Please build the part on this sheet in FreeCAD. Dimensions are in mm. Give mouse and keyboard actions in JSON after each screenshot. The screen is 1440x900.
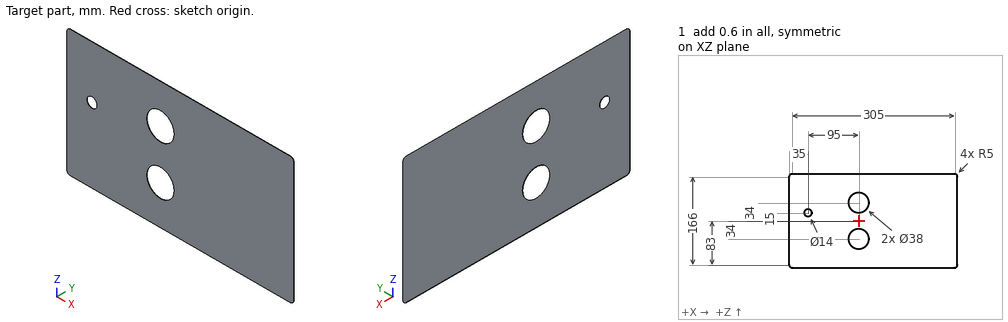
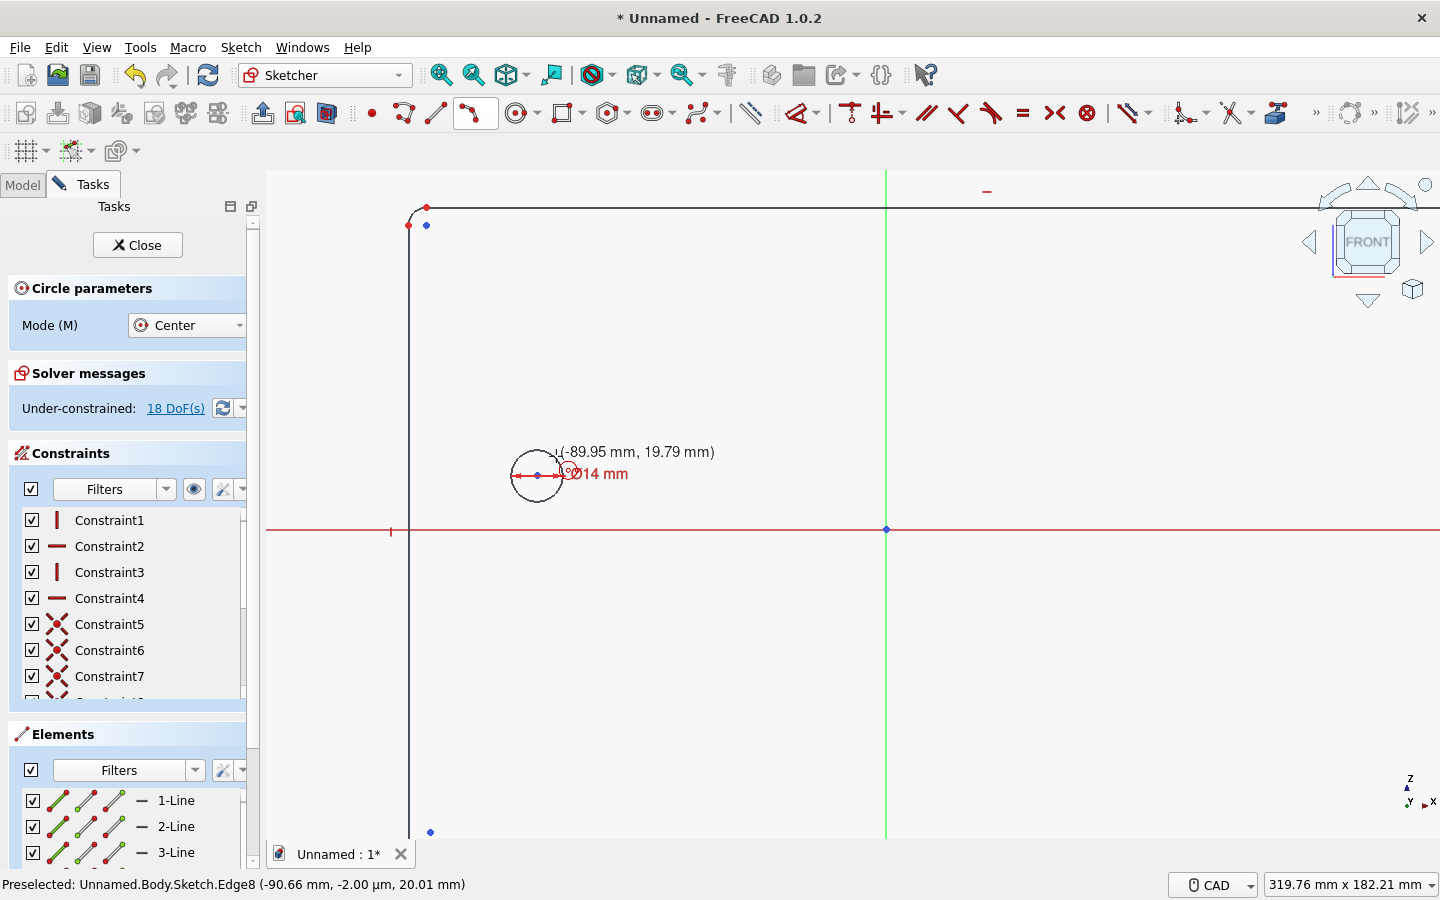
{"action": "left_click", "coordinate": [886, 405]}
{"action": "mouse_move", "coordinate": [936, 355]}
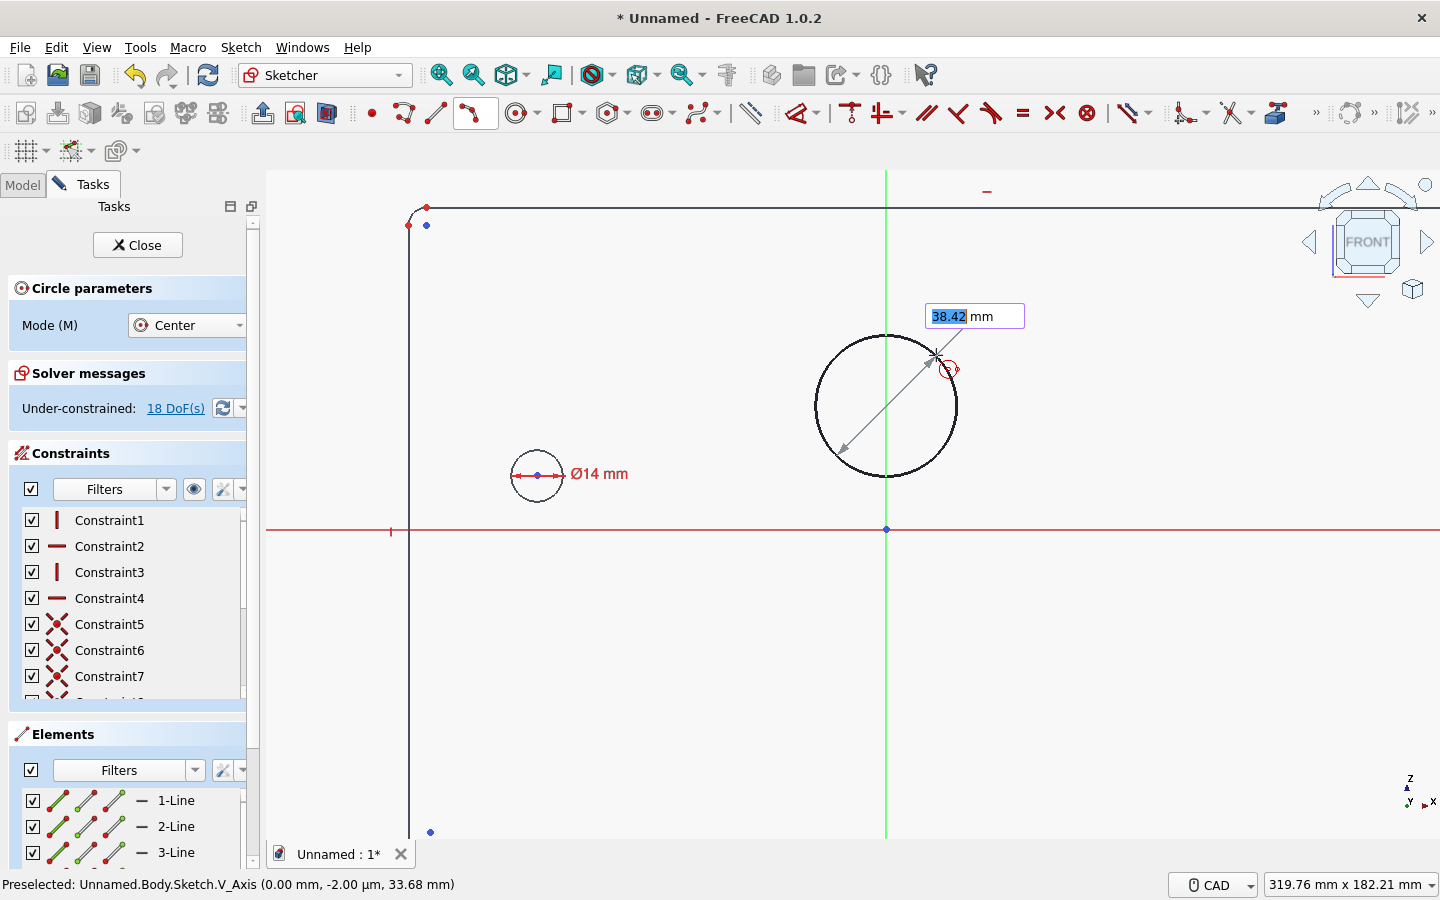
{"action": "type", "text": "38"}
{"action": "key", "text": "Return"}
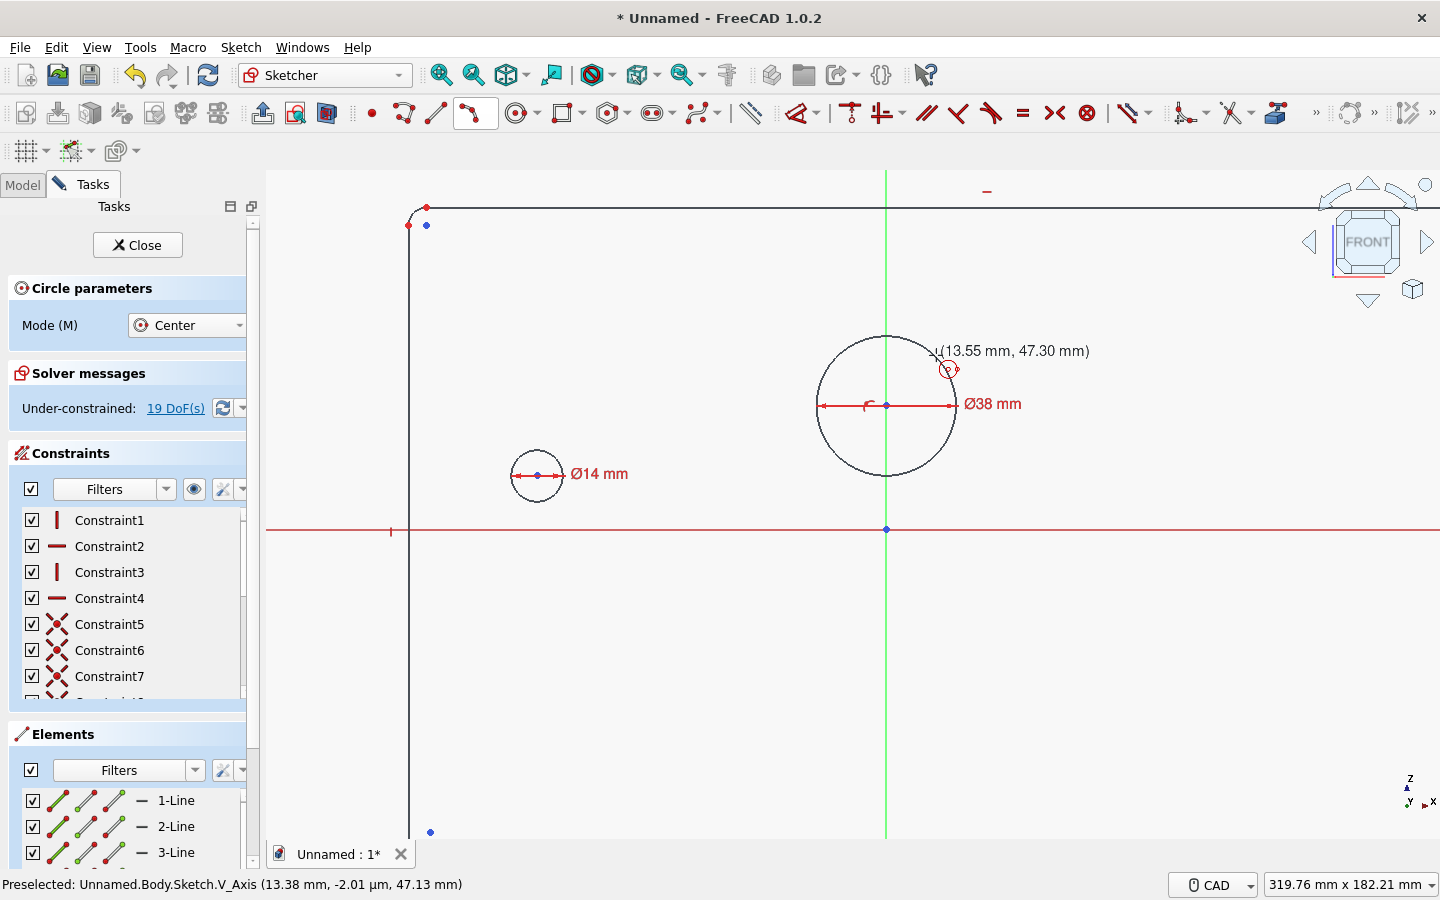
{"action": "left_click", "coordinate": [886, 654]}
{"action": "mouse_move", "coordinate": [936, 605]}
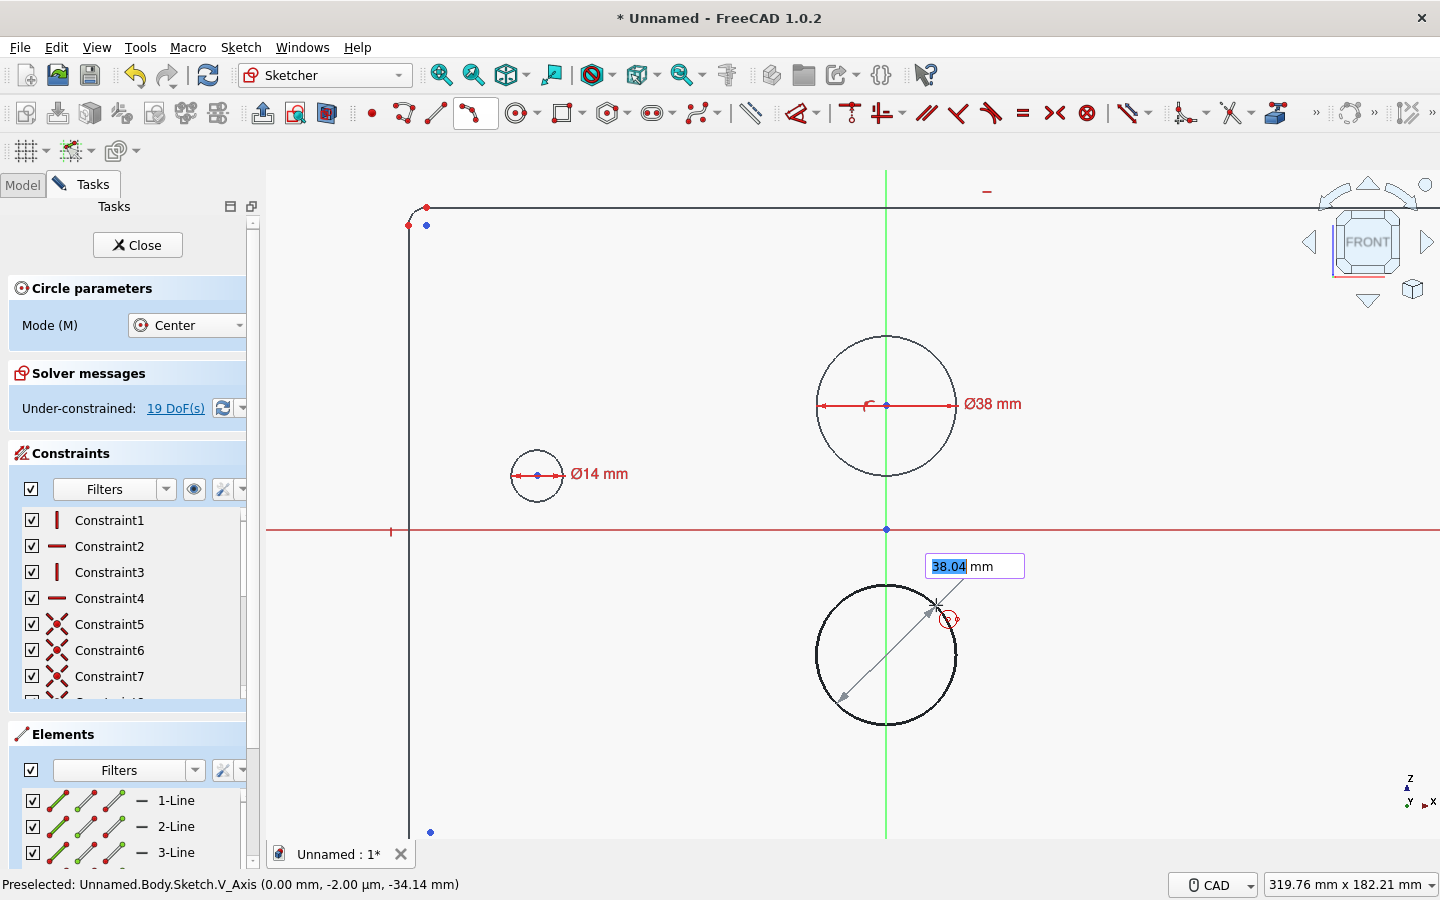
{"action": "type", "text": "38"}
{"action": "key", "text": "Return"}
{"action": "key", "text": "Escape"}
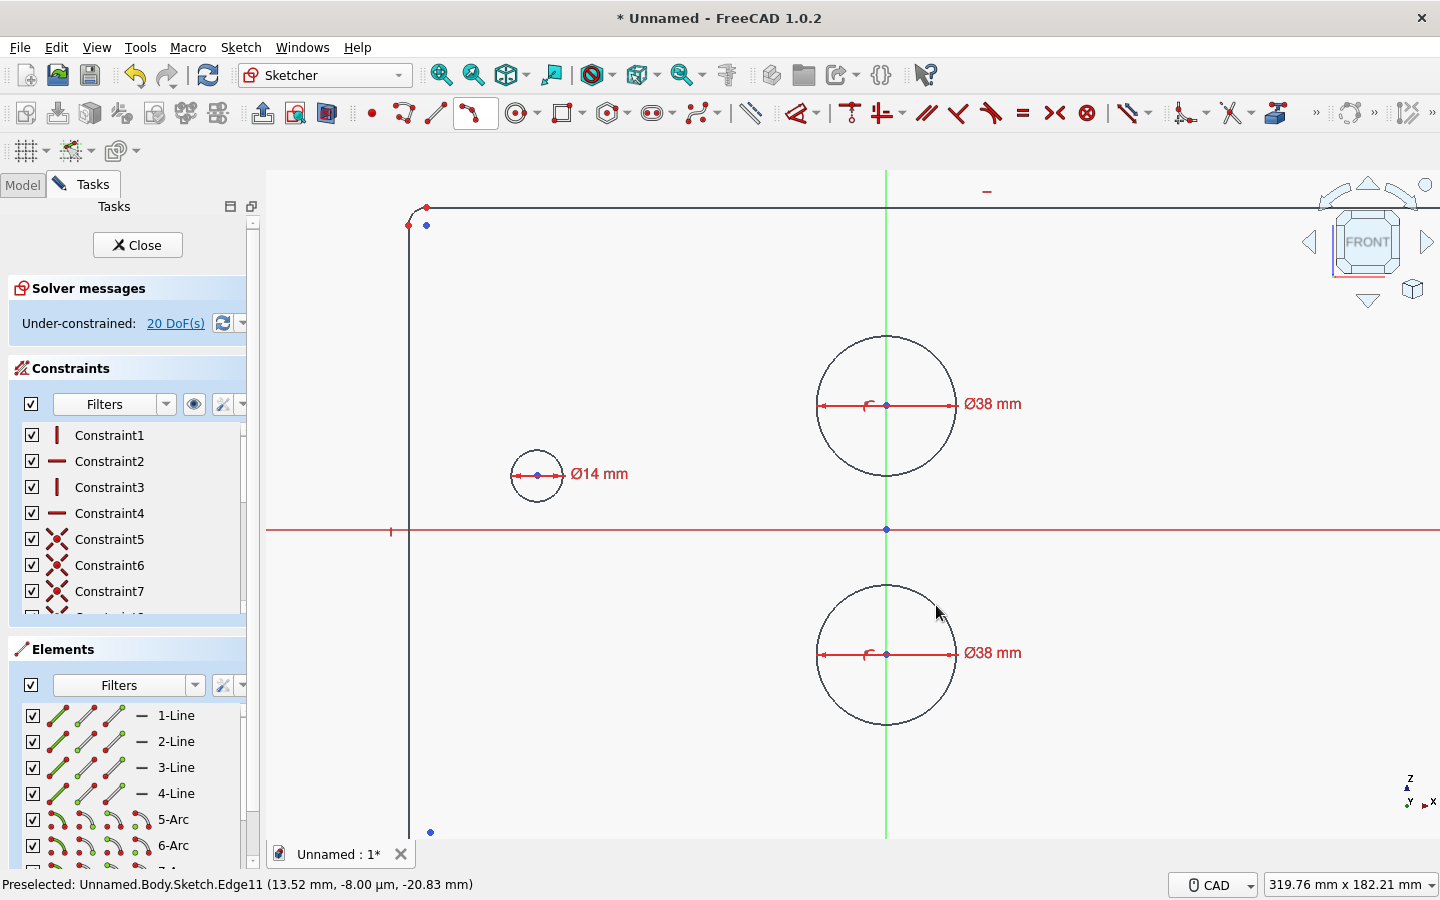
{"action": "left_click", "coordinate": [409, 653]}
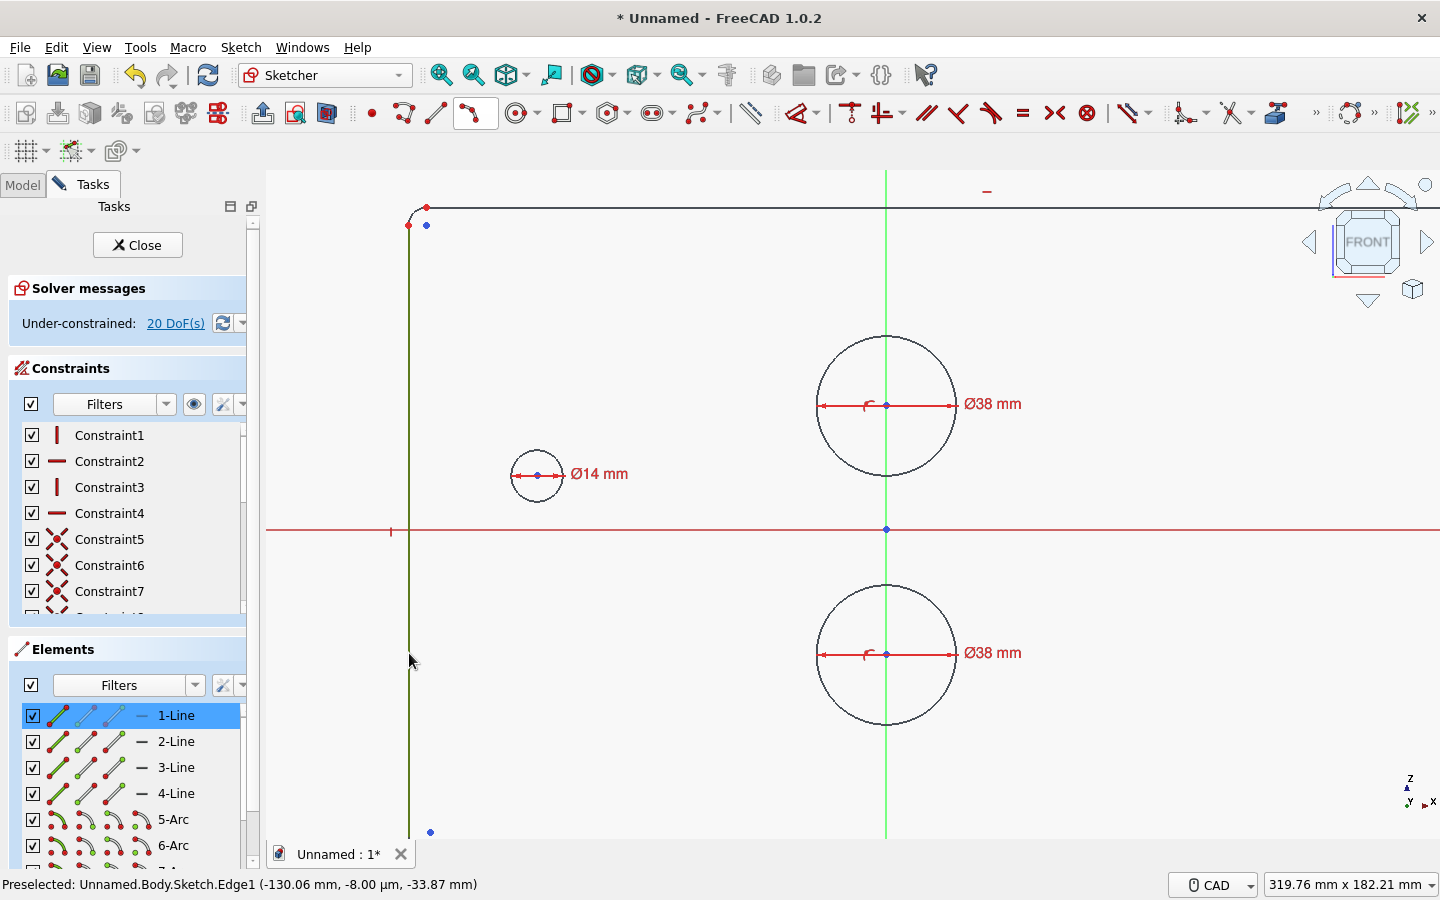
{"action": "left_click", "coordinate": [414, 213]}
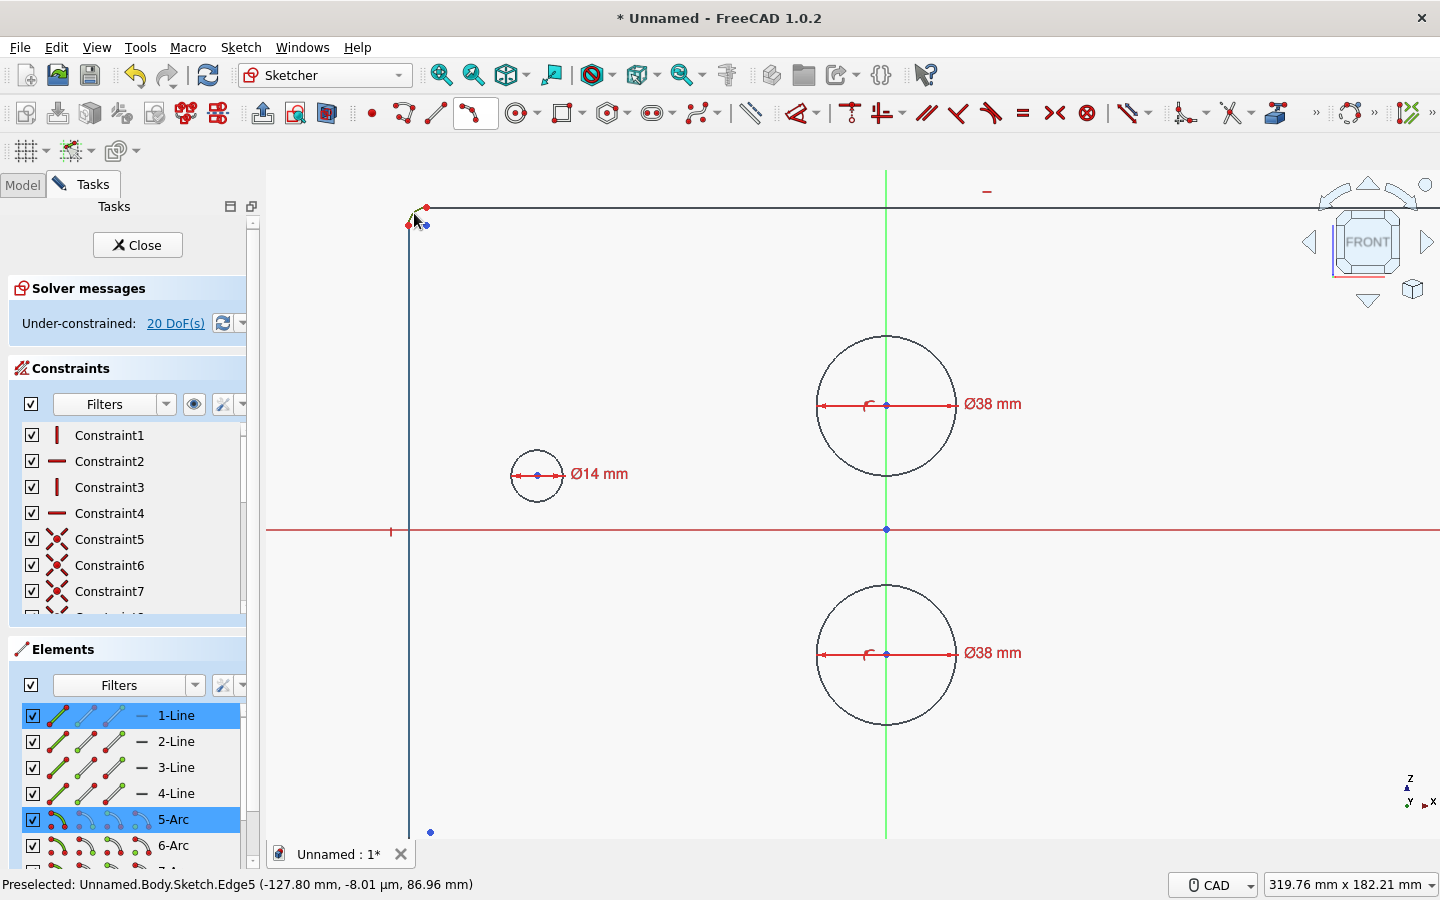
{"action": "left_click", "coordinate": [992, 114]}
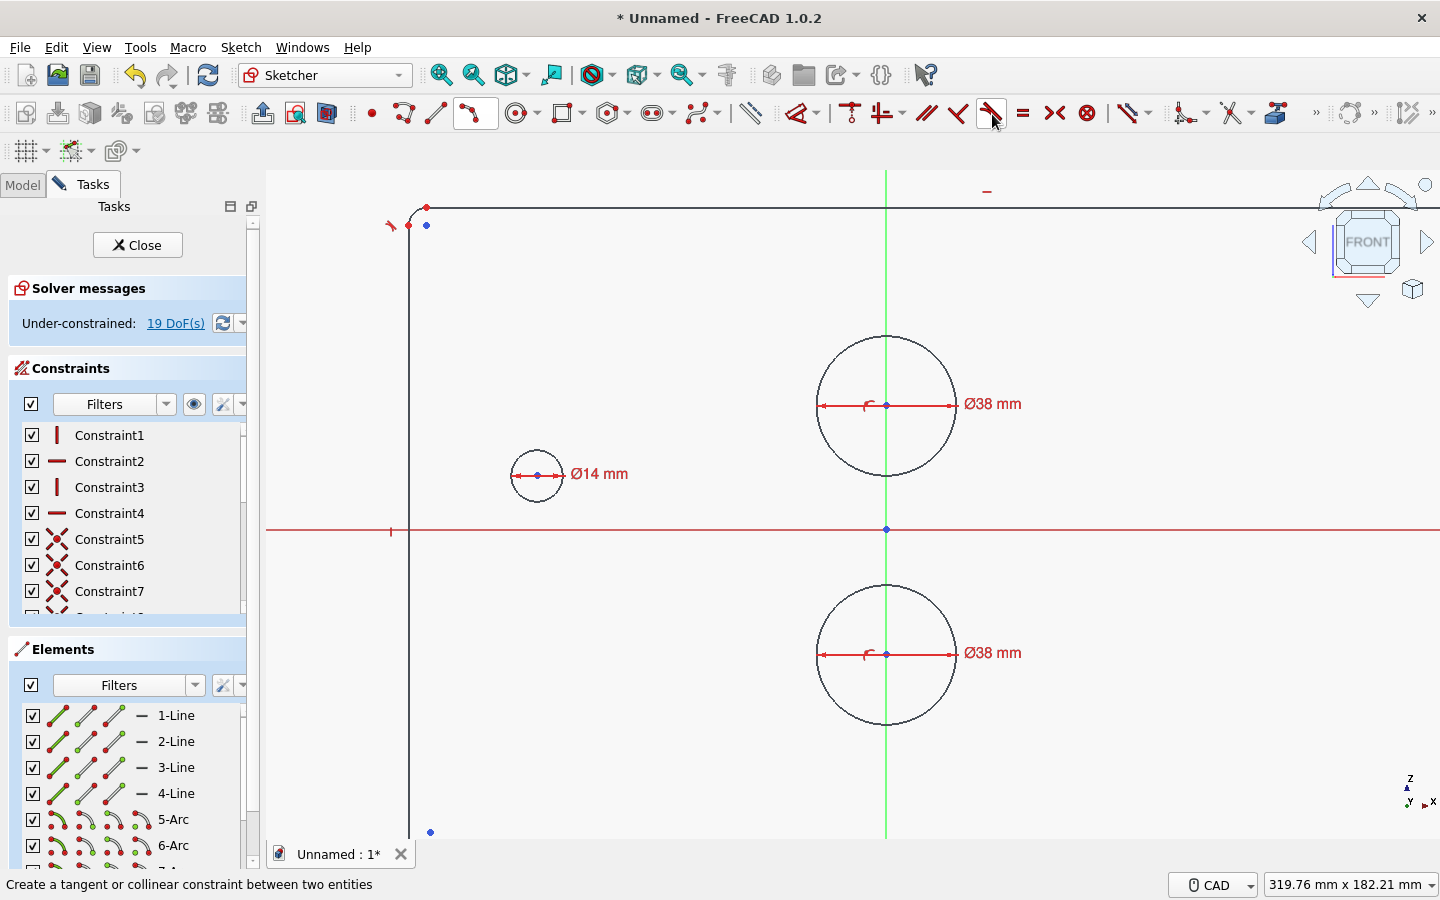
{"action": "left_click", "coordinate": [409, 653]}